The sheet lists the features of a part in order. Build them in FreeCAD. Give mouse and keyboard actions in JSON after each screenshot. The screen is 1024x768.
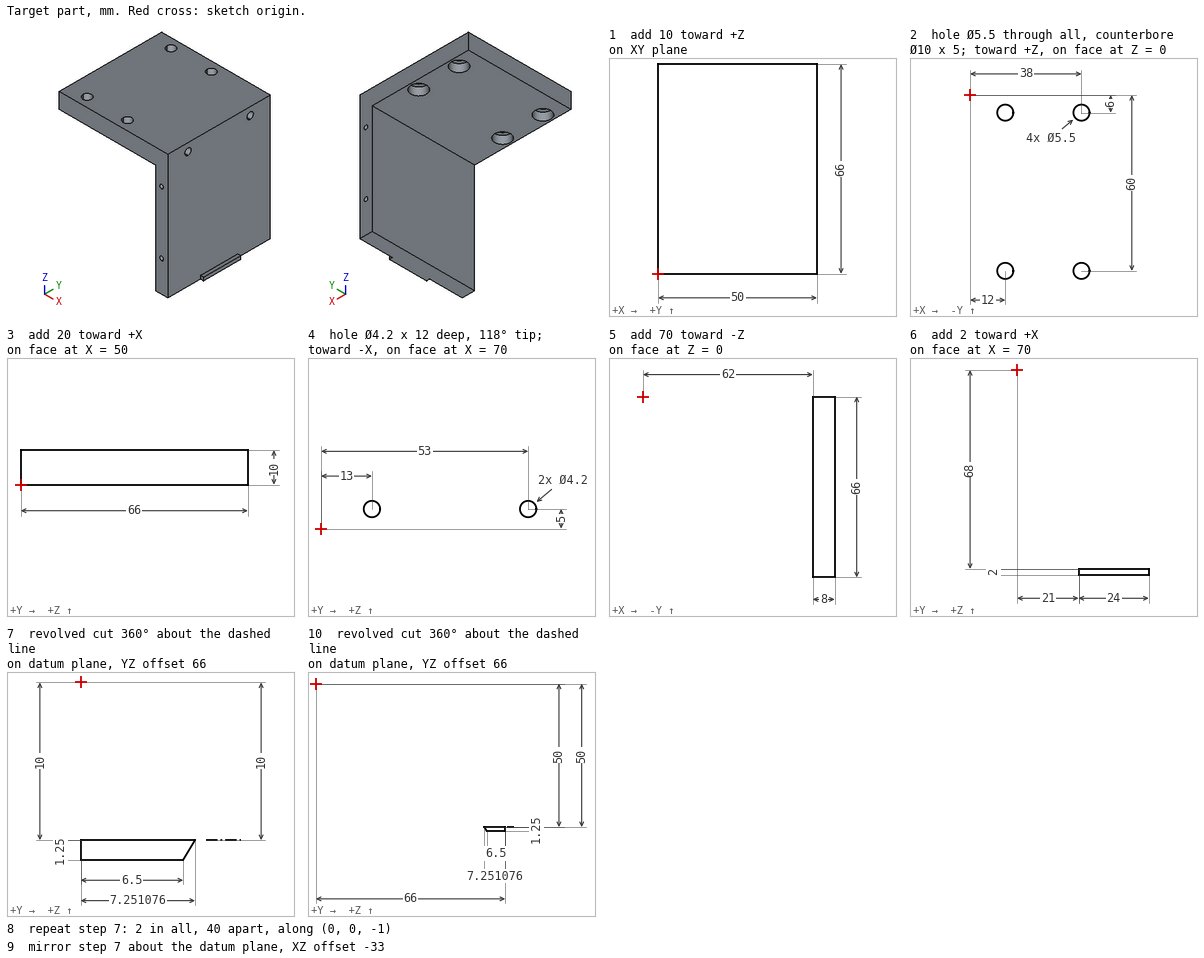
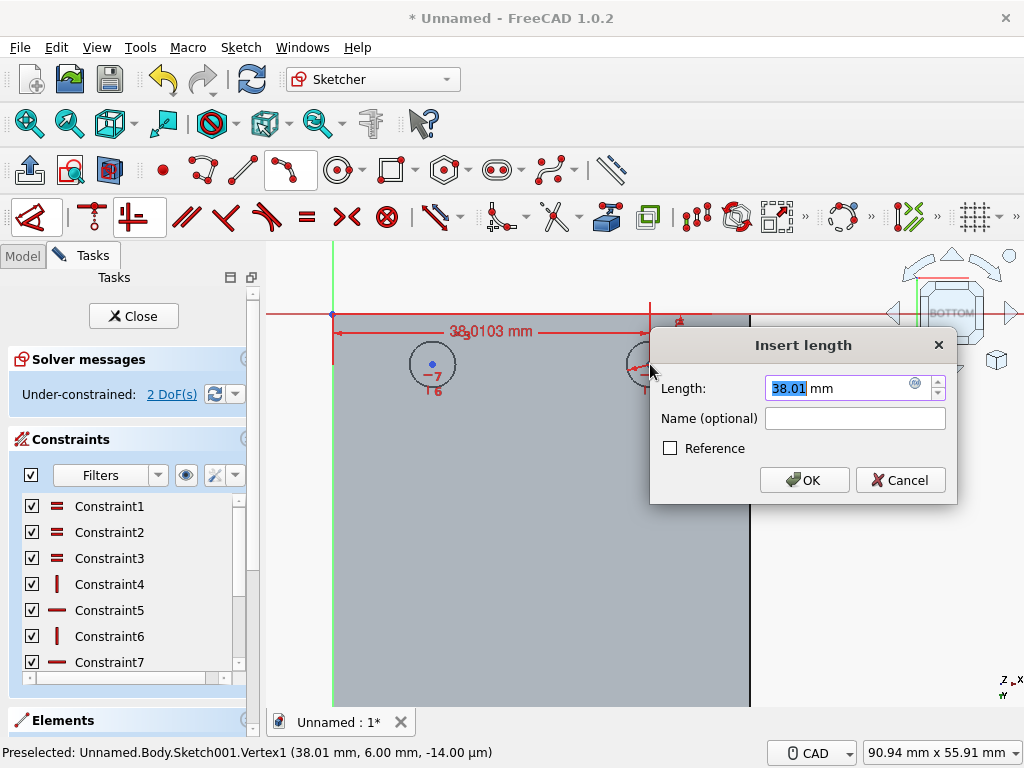
{"action": "type", "text": "38"}
{"action": "key", "text": "Return"}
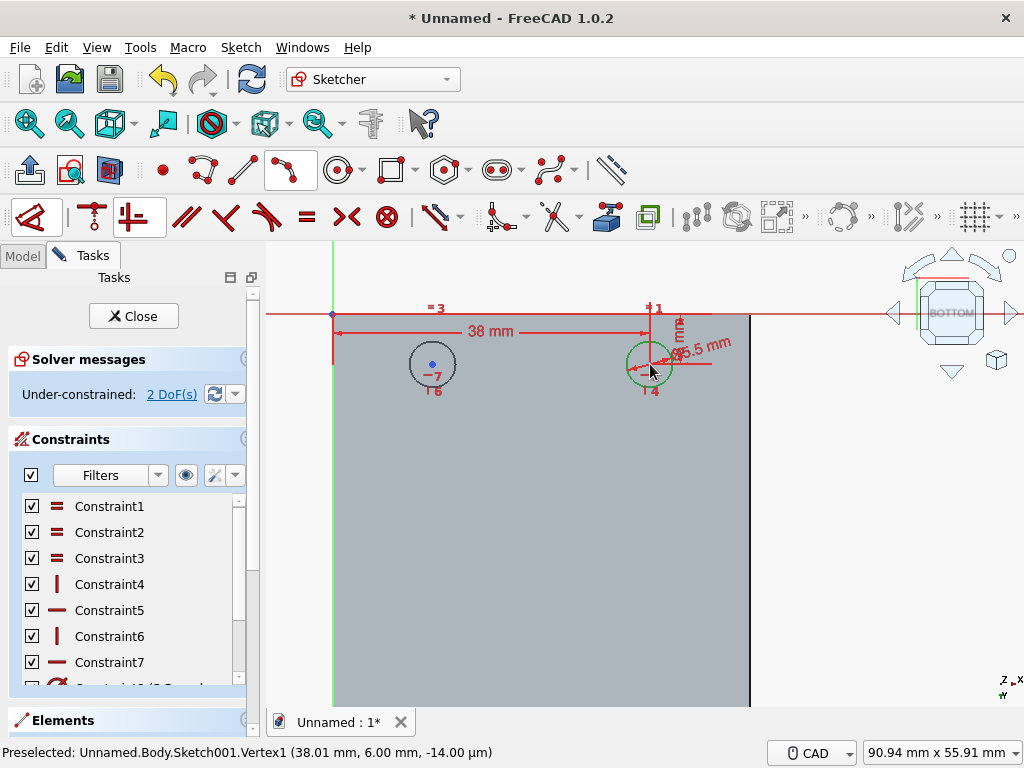
{"action": "scroll", "coordinate": [666, 350], "scroll_direction": "down", "scroll_amount": 3}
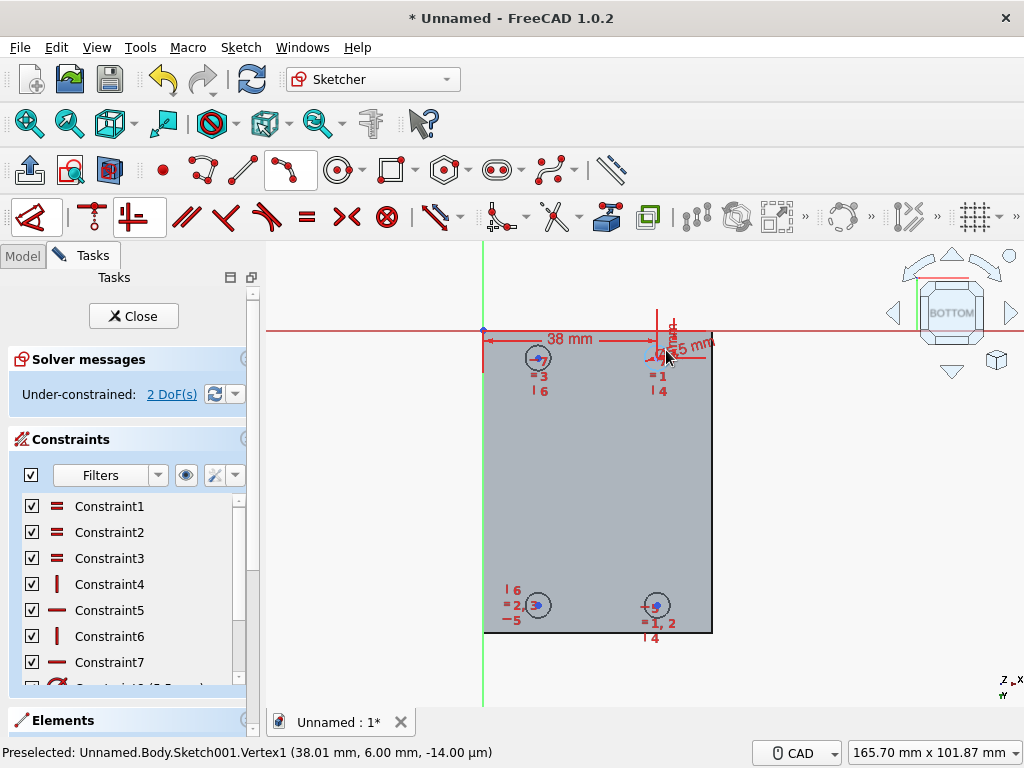
{"action": "left_click", "coordinate": [657, 605]}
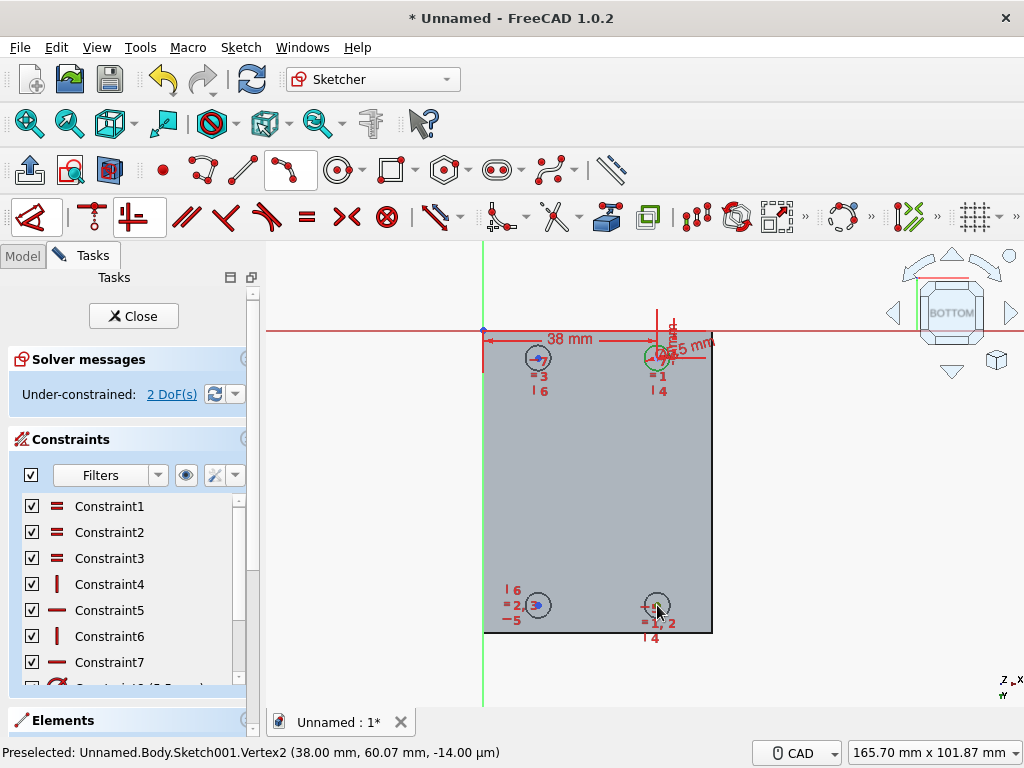
{"action": "left_click", "coordinate": [56, 218]}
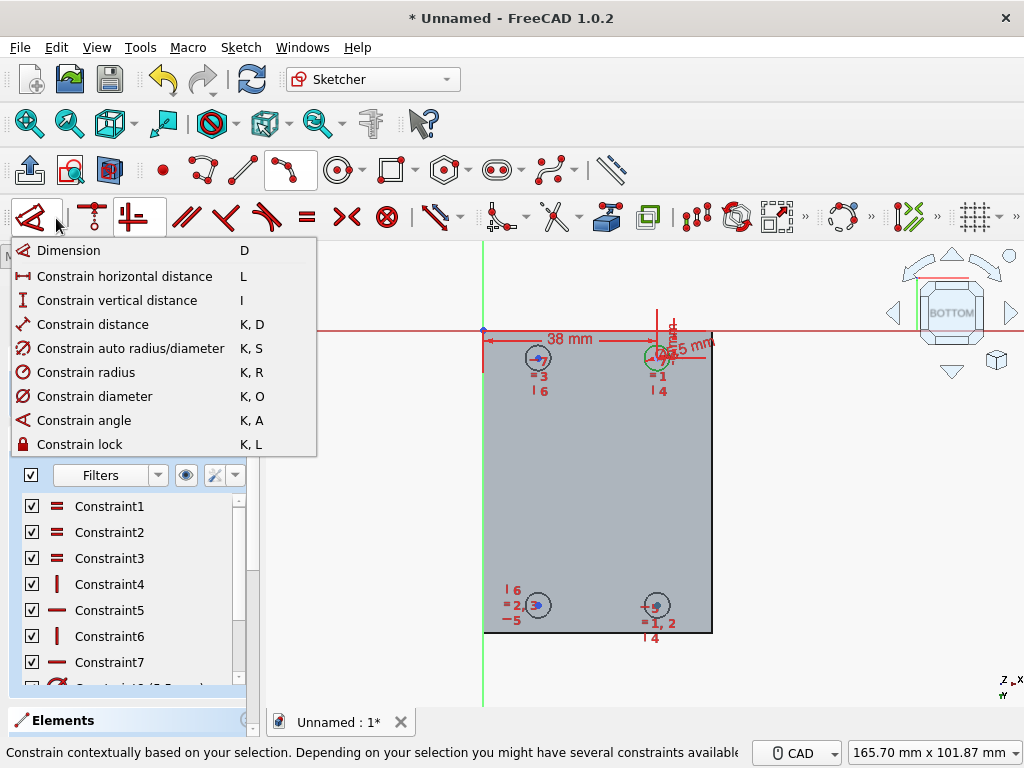
{"action": "left_click", "coordinate": [164, 300]}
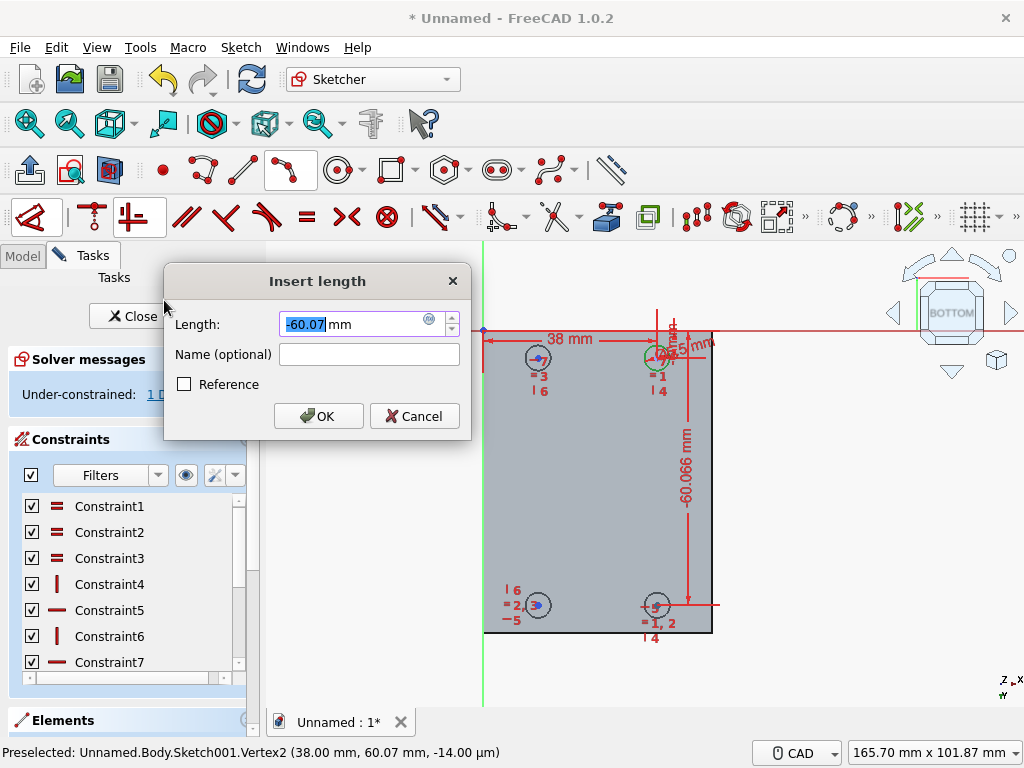
{"action": "type", "text": "-60"}
{"action": "key", "text": "Return"}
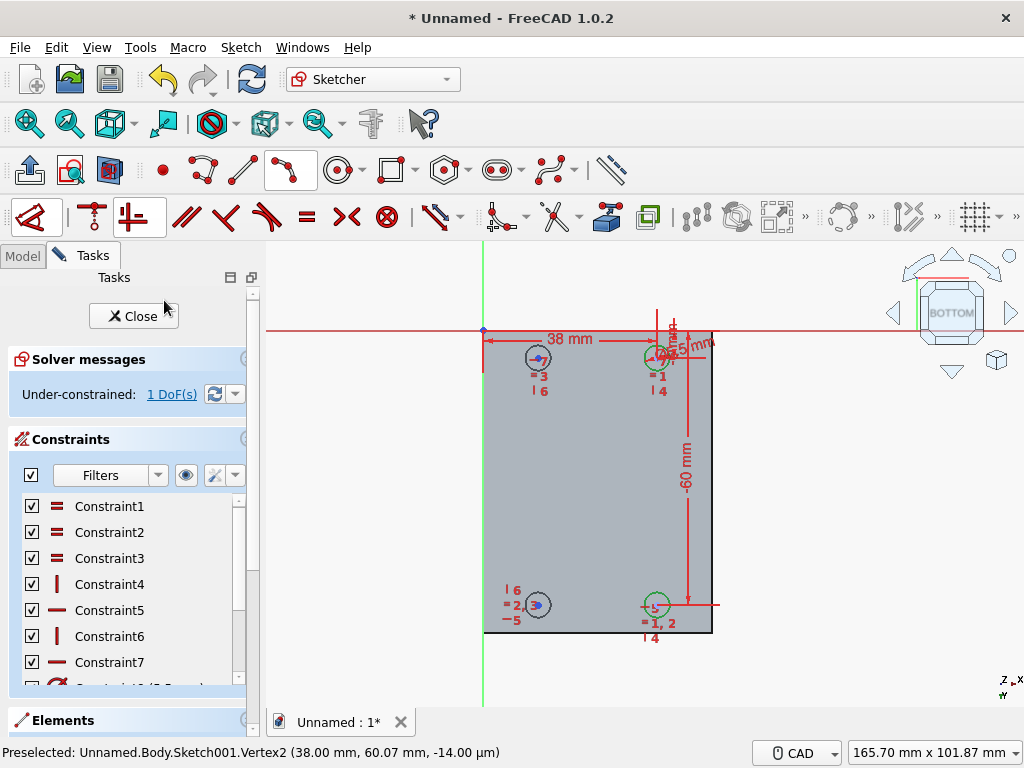
{"action": "left_click", "coordinate": [538, 605]}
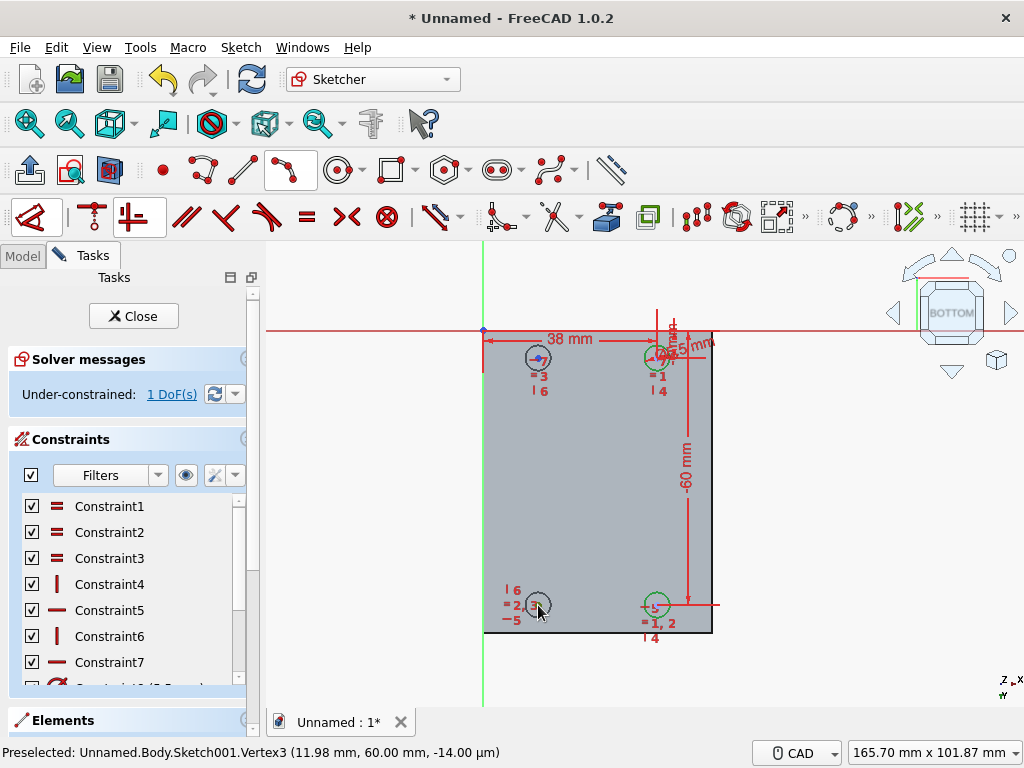
{"action": "key", "text": "l"}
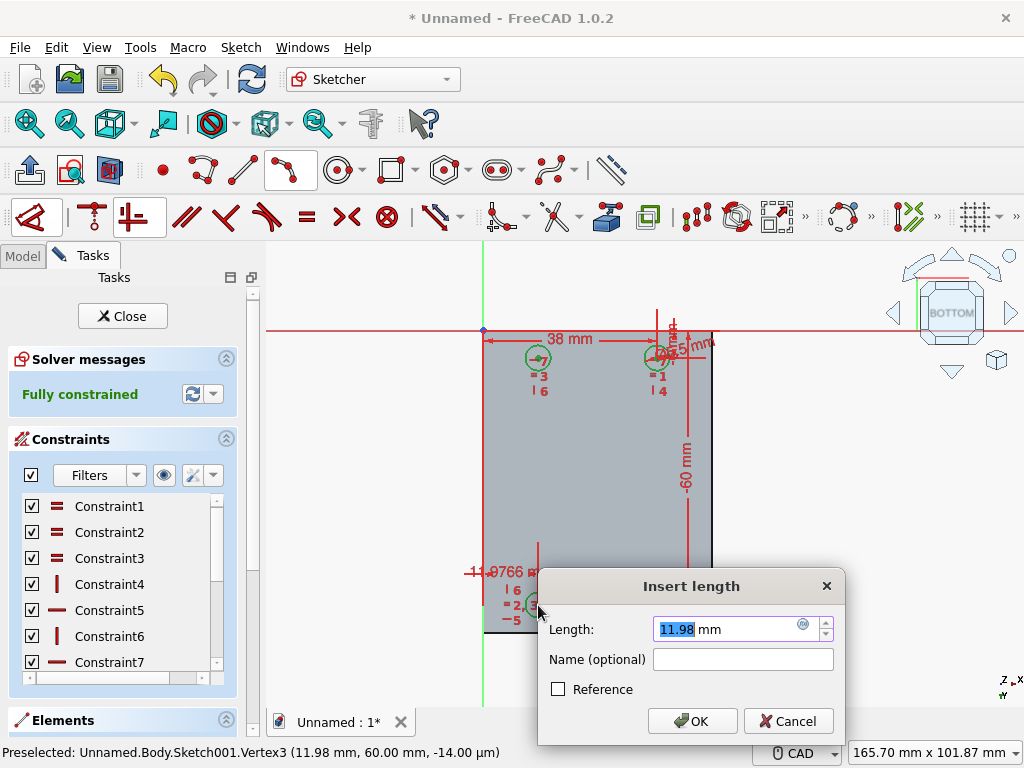
{"action": "type", "text": "12"}
{"action": "key", "text": "Return"}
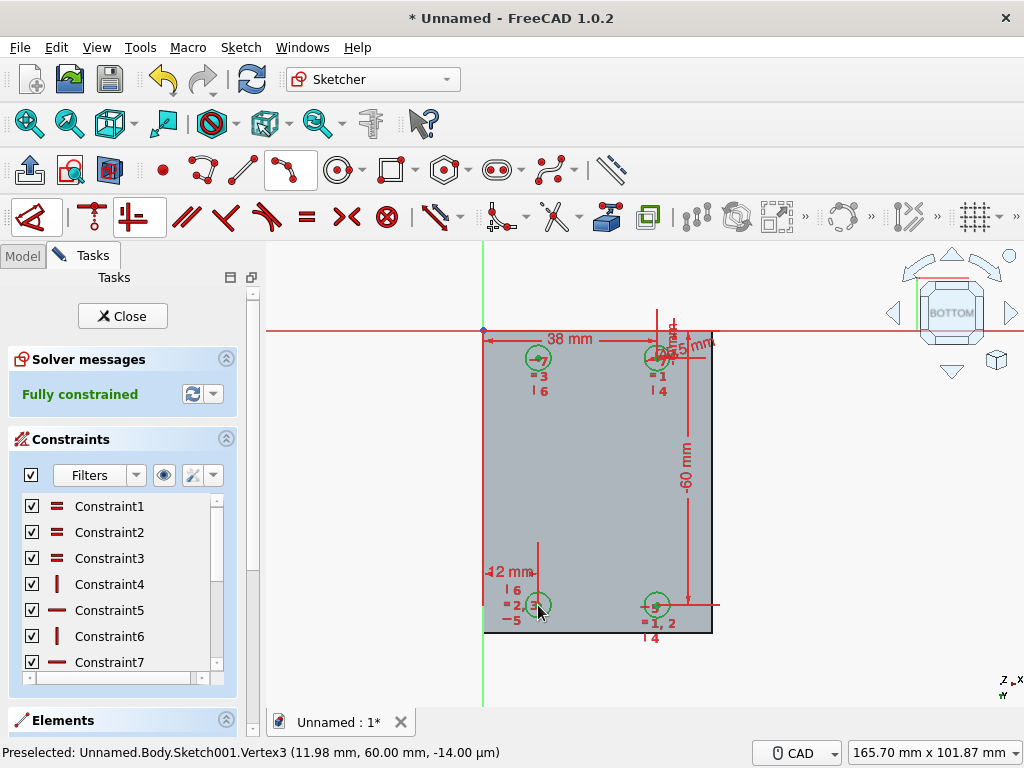
{"action": "left_click", "coordinate": [123, 316]}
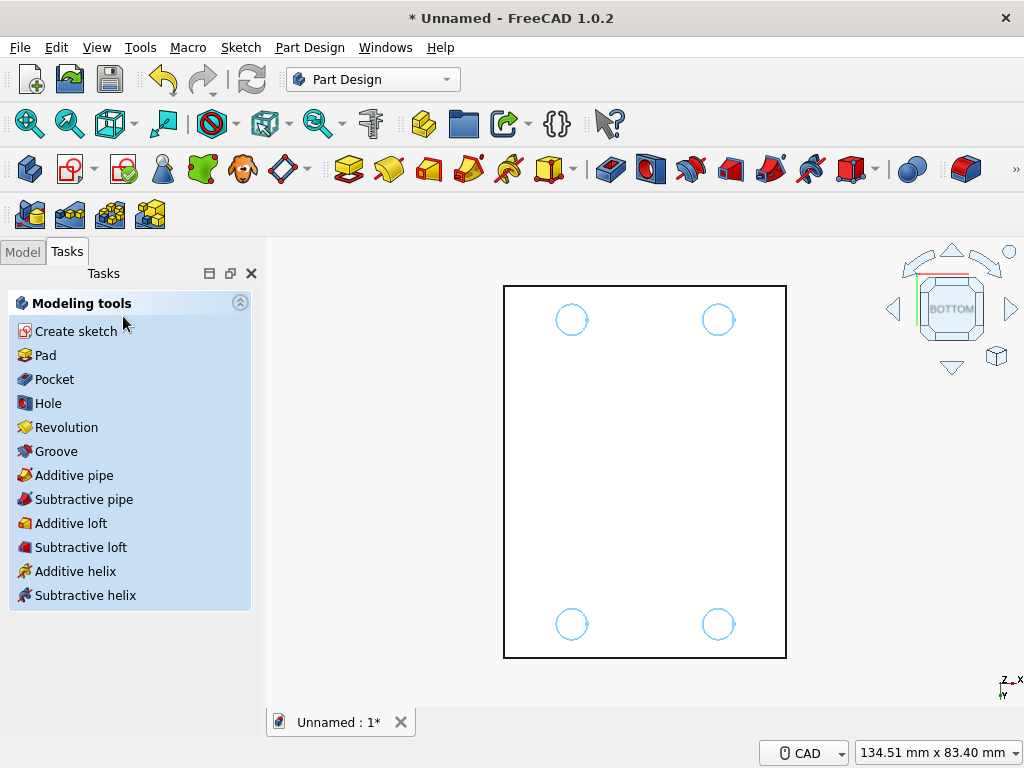
{"action": "left_click", "coordinate": [652, 170]}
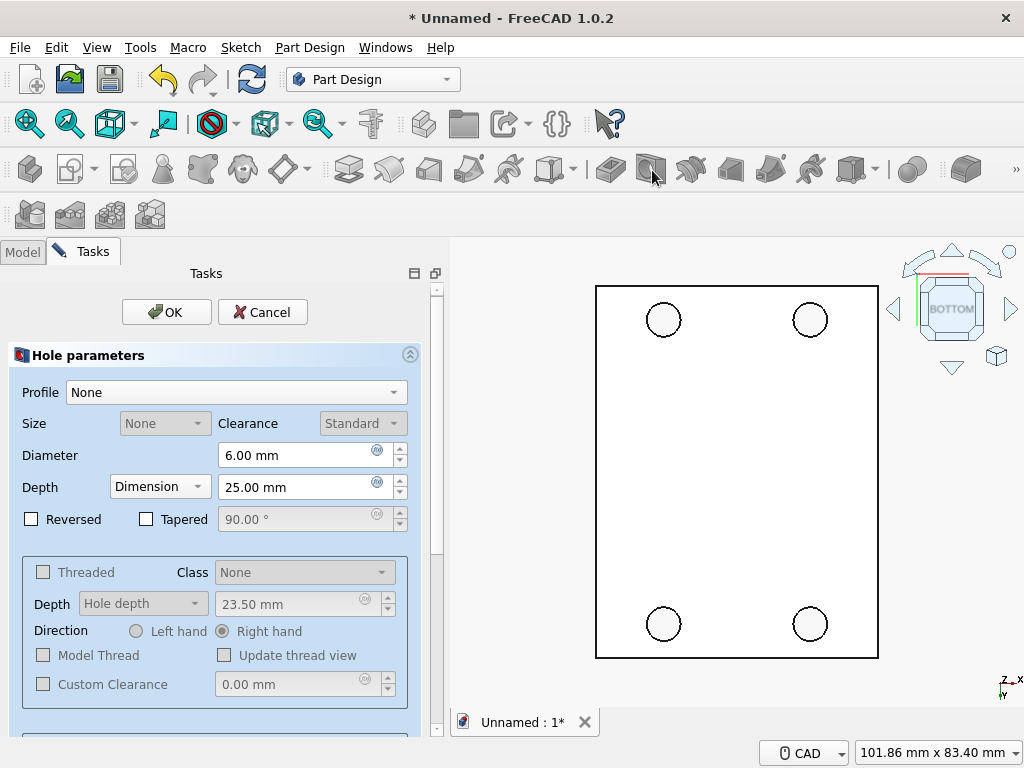
{"action": "triple_click", "coordinate": [305, 455]}